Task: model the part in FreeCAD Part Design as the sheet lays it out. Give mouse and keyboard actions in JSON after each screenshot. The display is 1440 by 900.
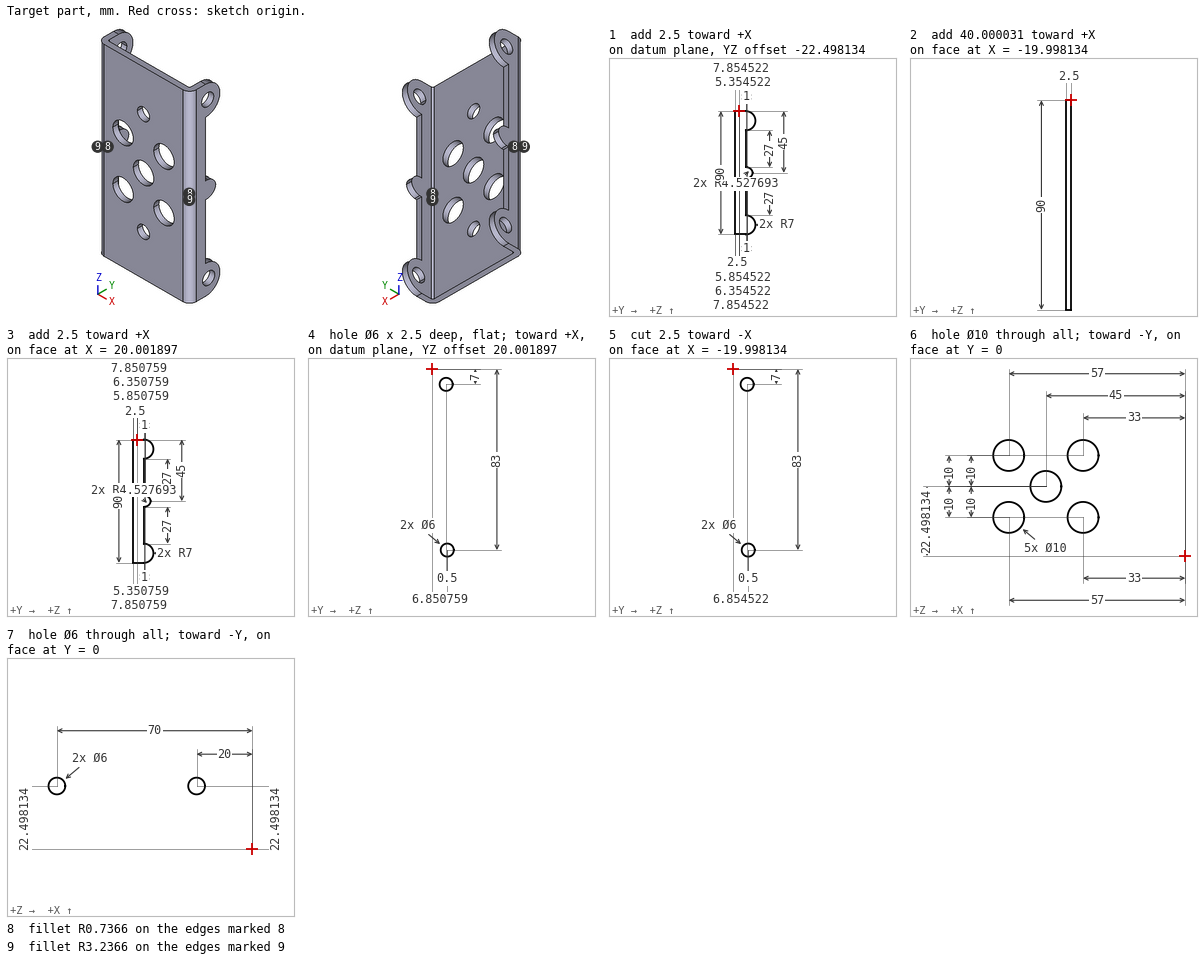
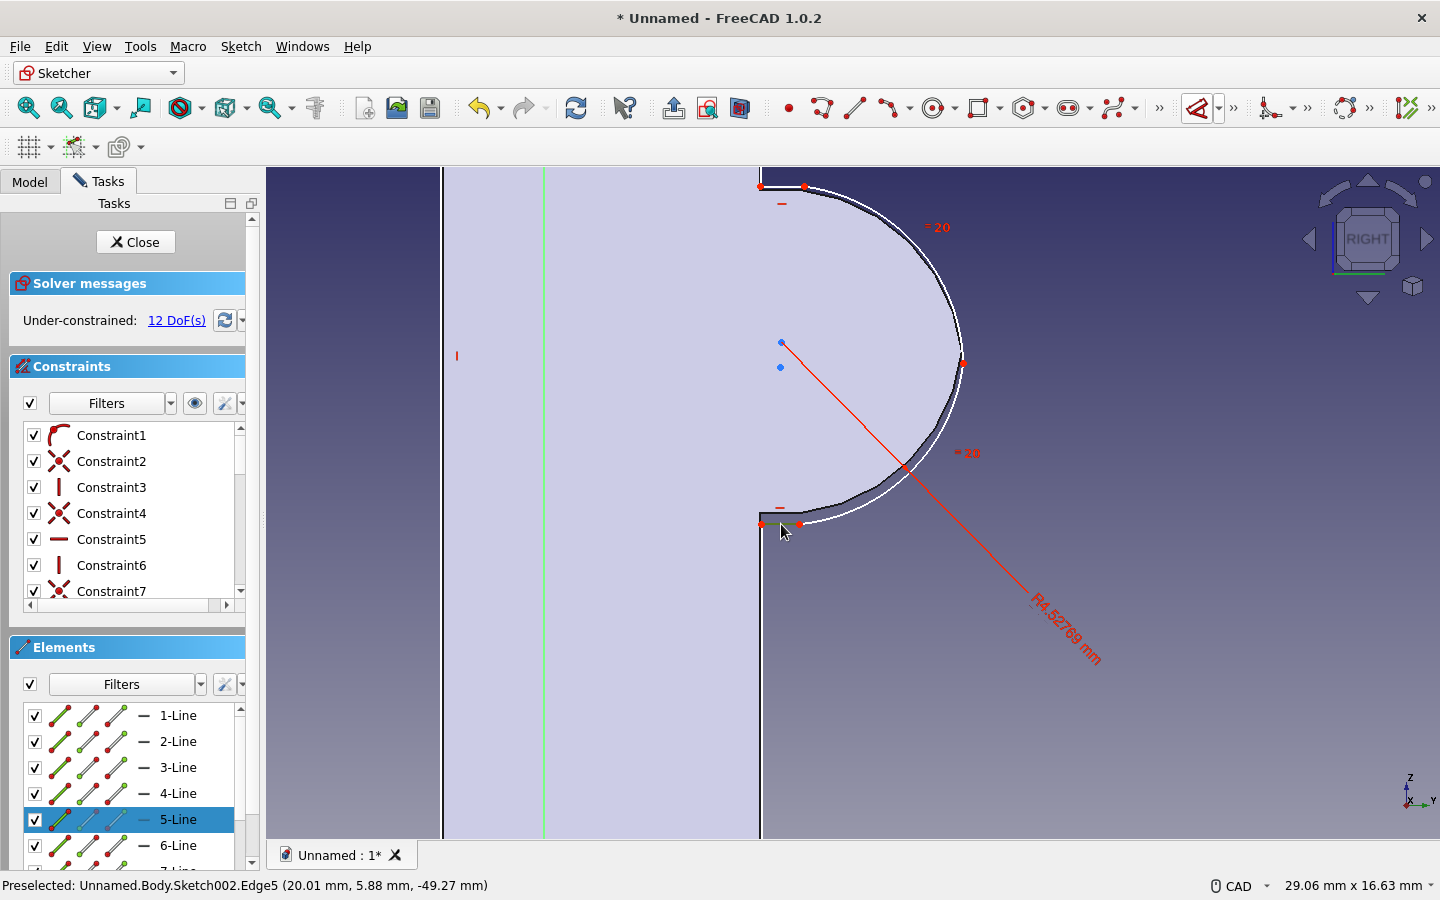
{"action": "key", "text": "l"}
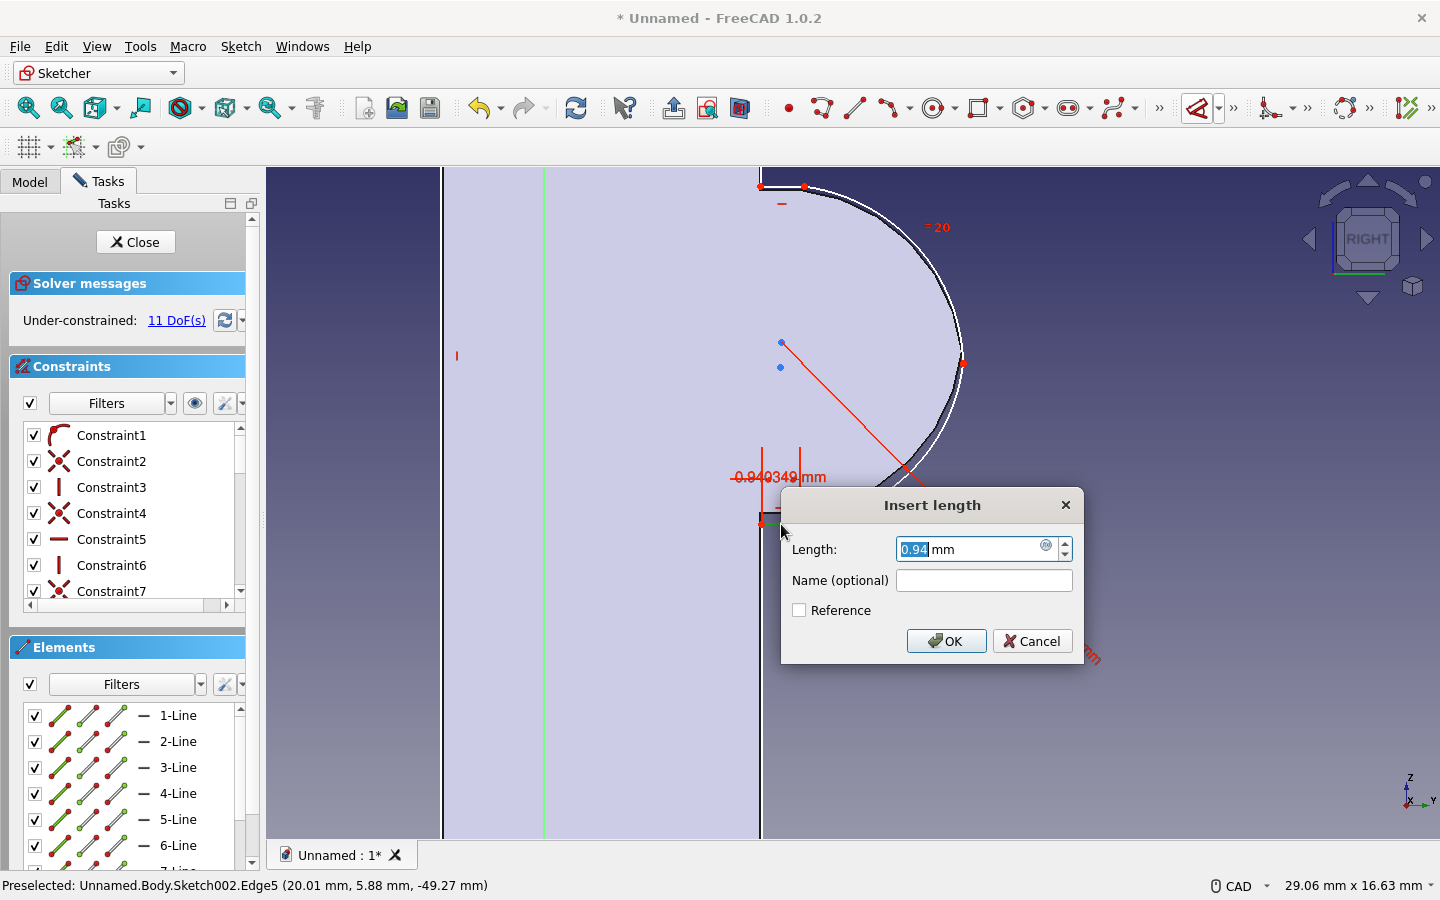
{"action": "type", "text": "1"}
{"action": "key", "text": "Return"}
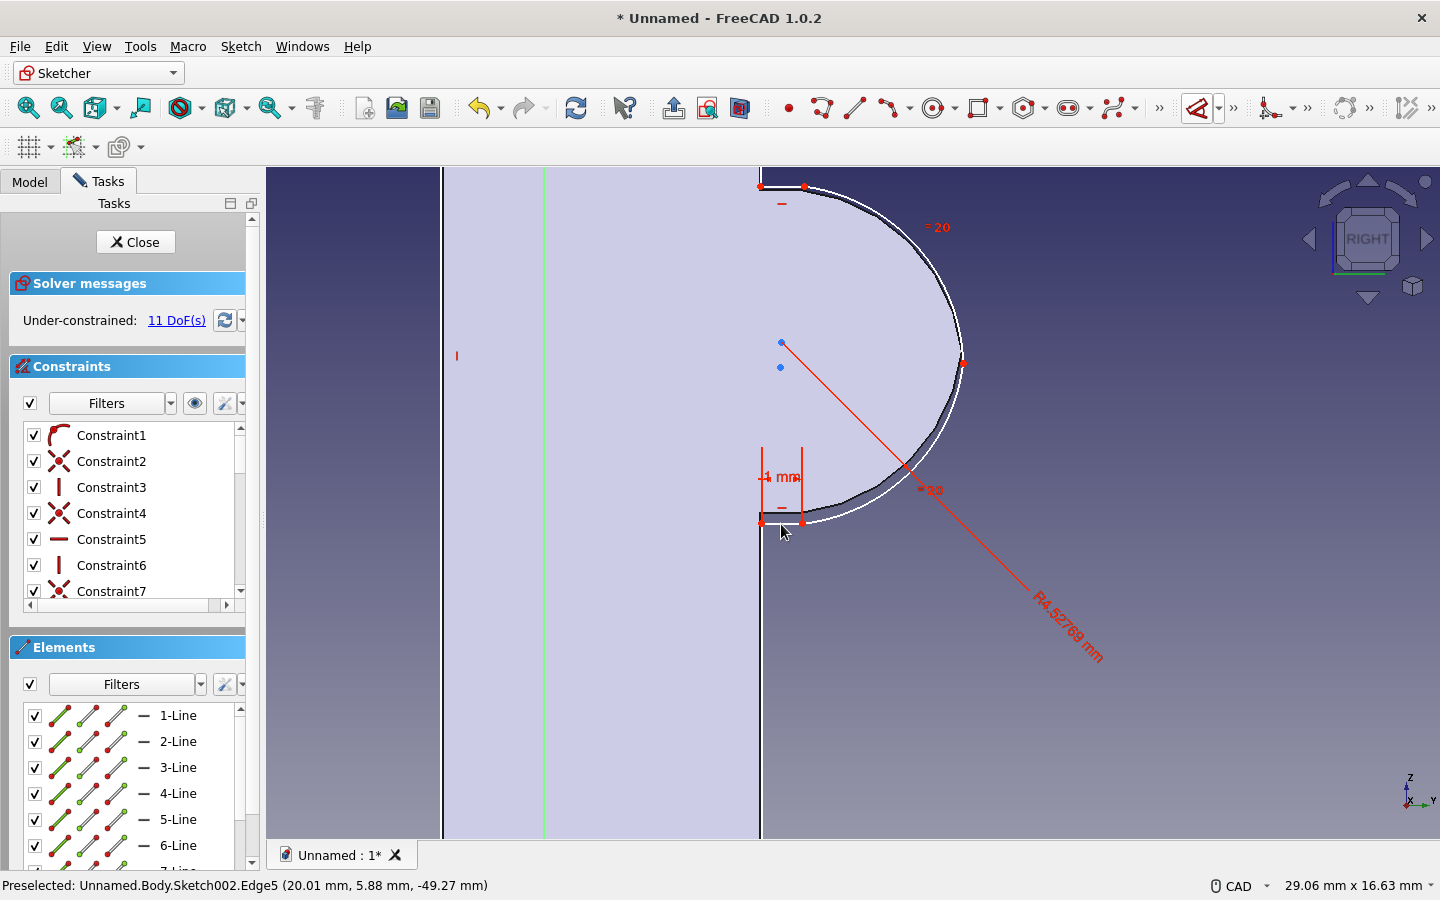
{"action": "scroll", "coordinate": [790, 522], "scroll_direction": "down", "scroll_amount": 11}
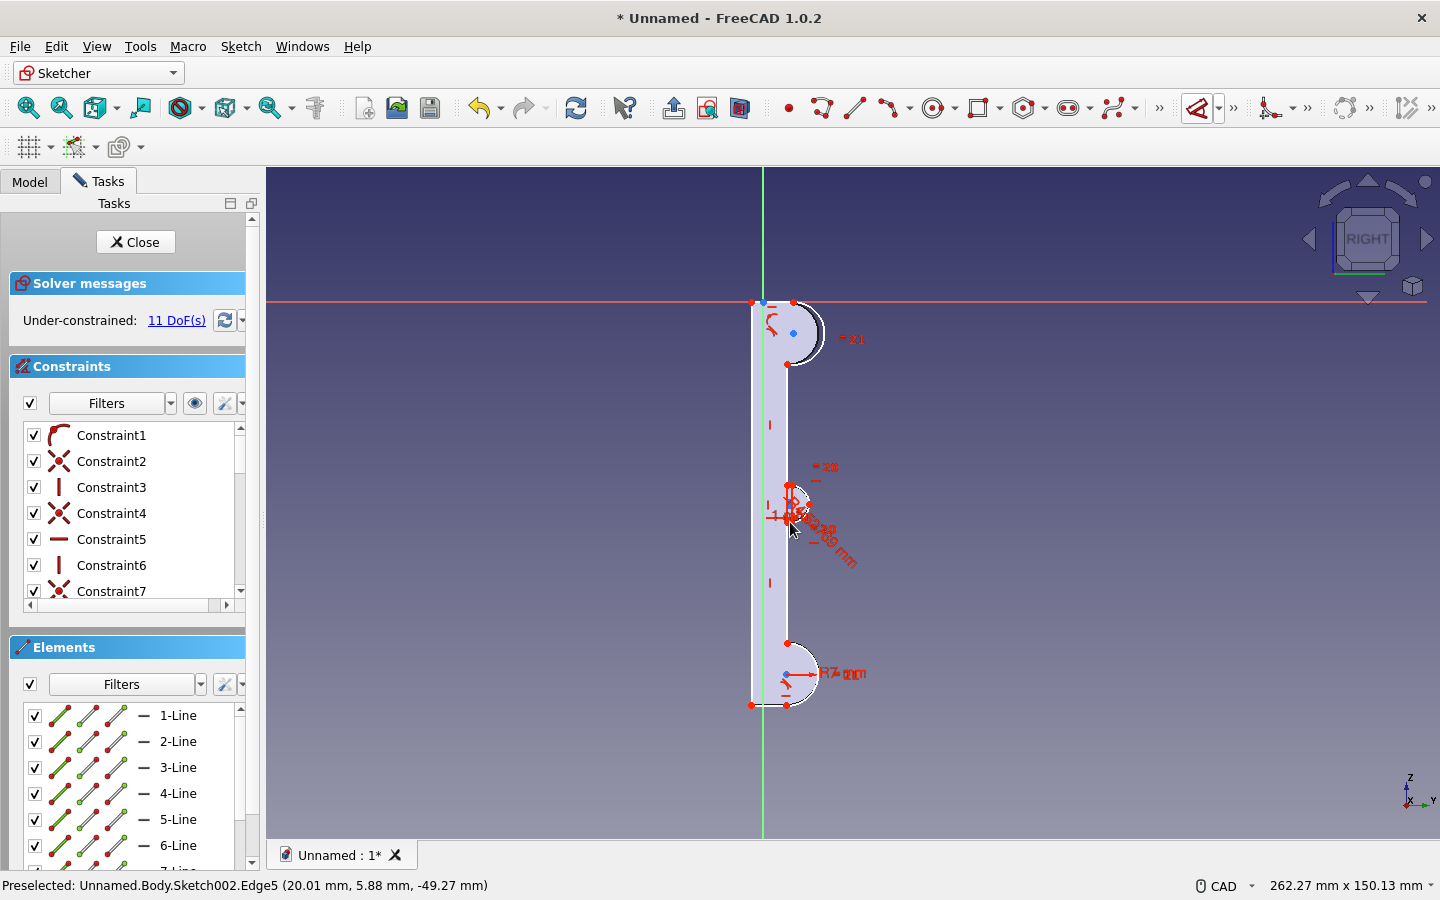
{"action": "scroll", "coordinate": [791, 485], "scroll_direction": "up", "scroll_amount": 12}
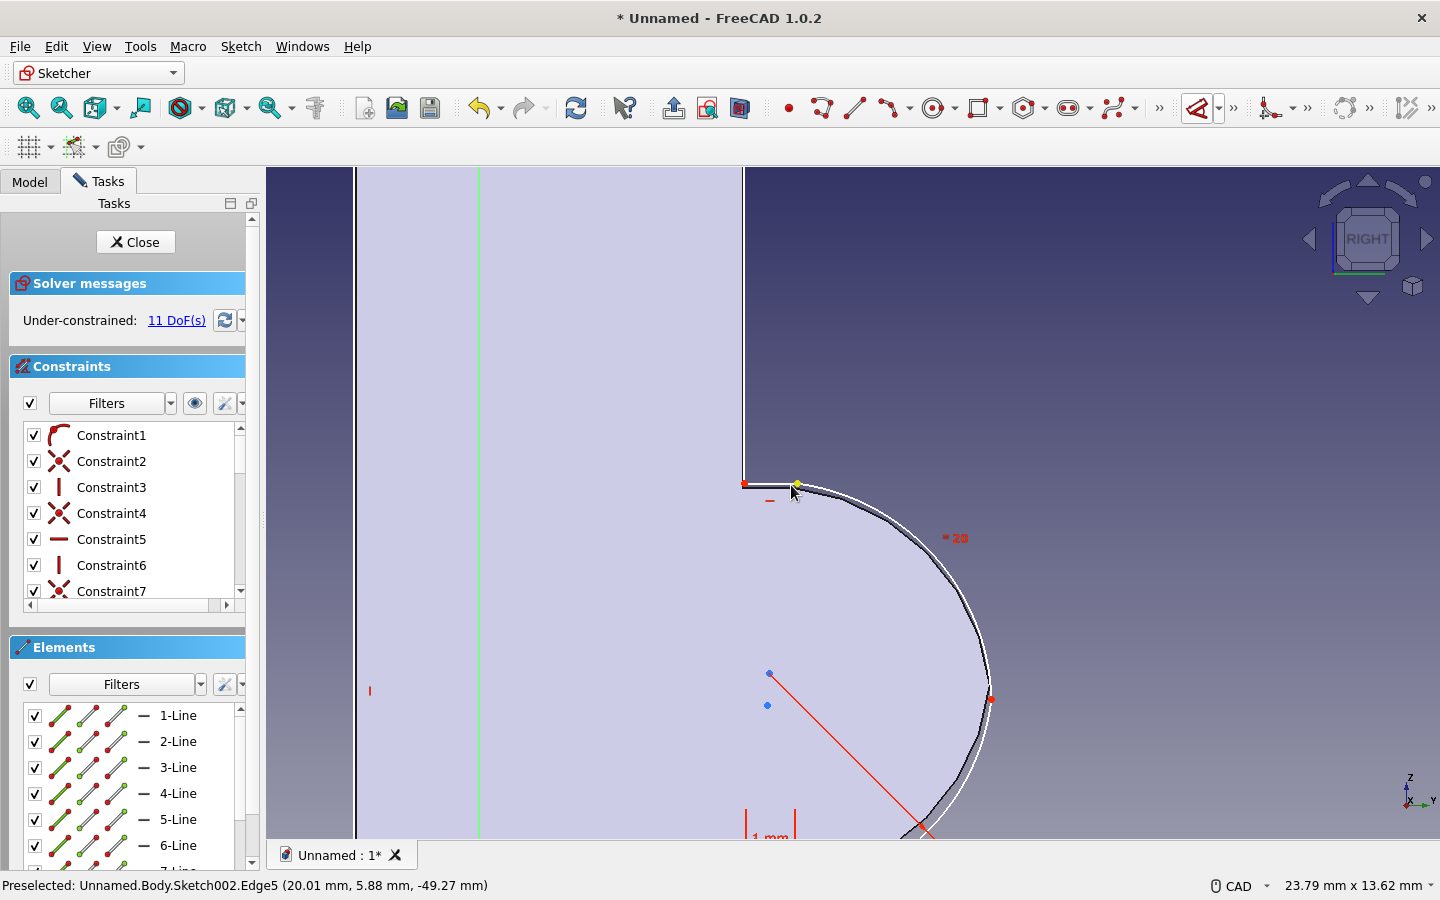
{"action": "left_click", "coordinate": [782, 484]}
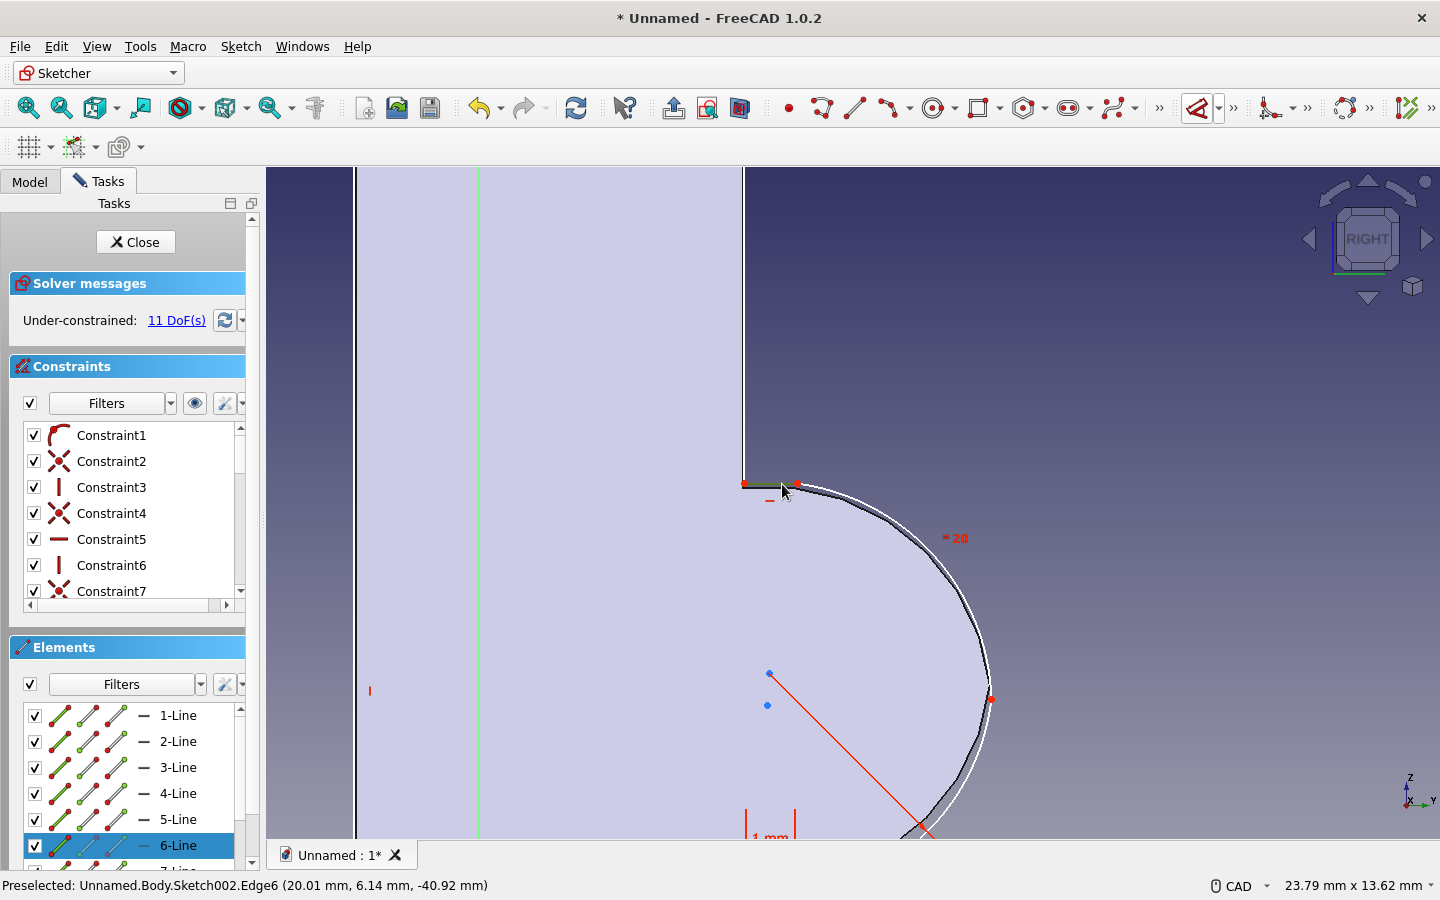
{"action": "key", "text": "l"}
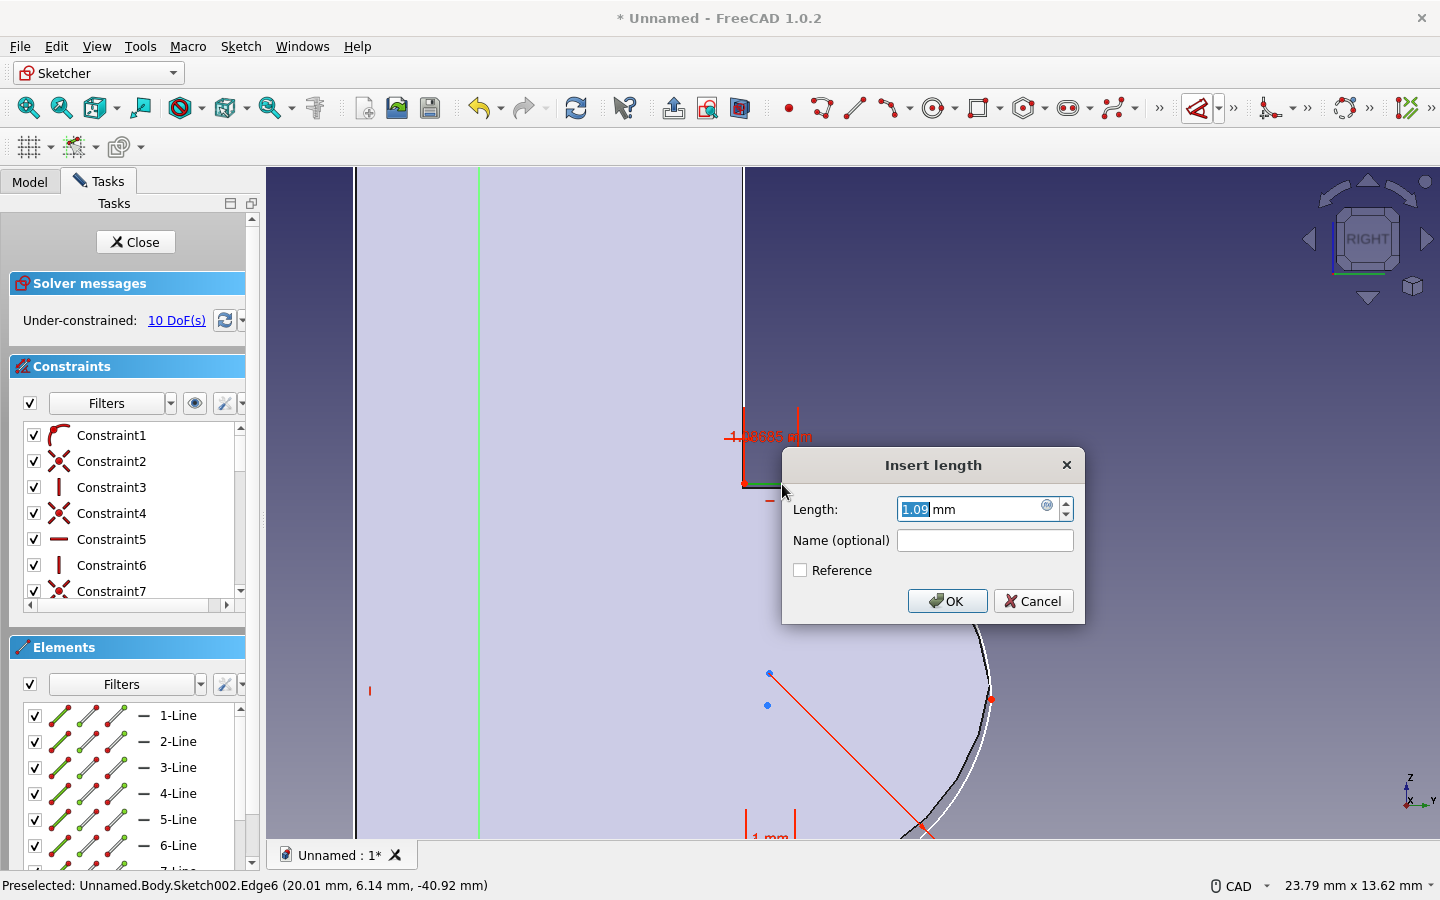
{"action": "type", "text": "1"}
{"action": "key", "text": "Return"}